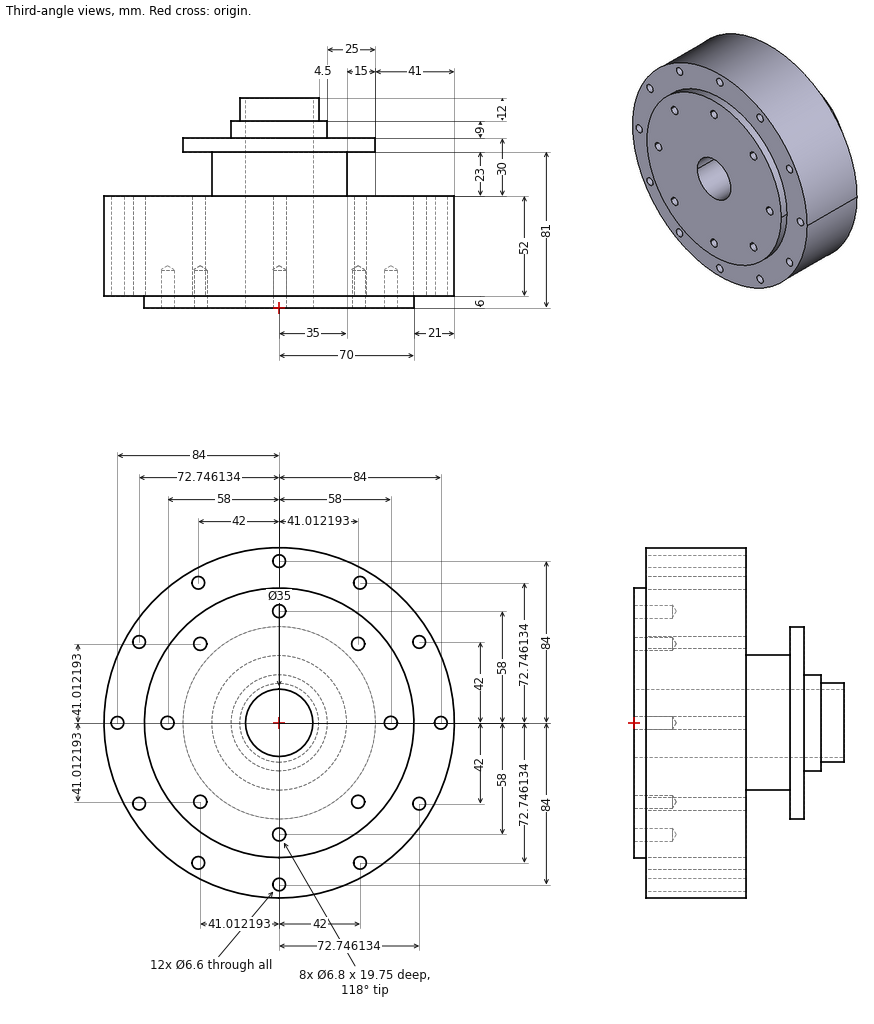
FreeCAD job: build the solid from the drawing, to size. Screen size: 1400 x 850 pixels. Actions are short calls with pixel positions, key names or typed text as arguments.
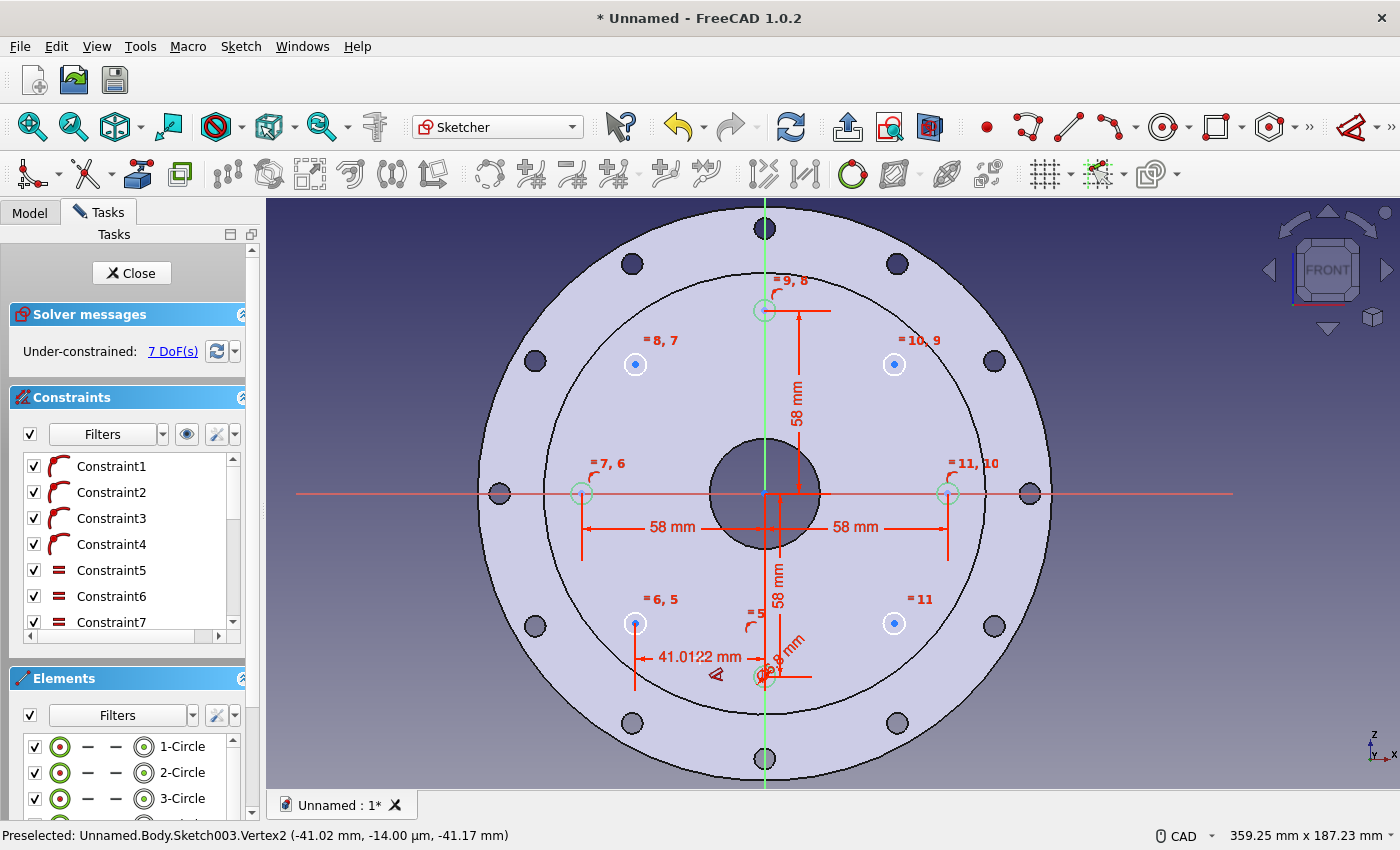
click(635, 624)
click(601, 559)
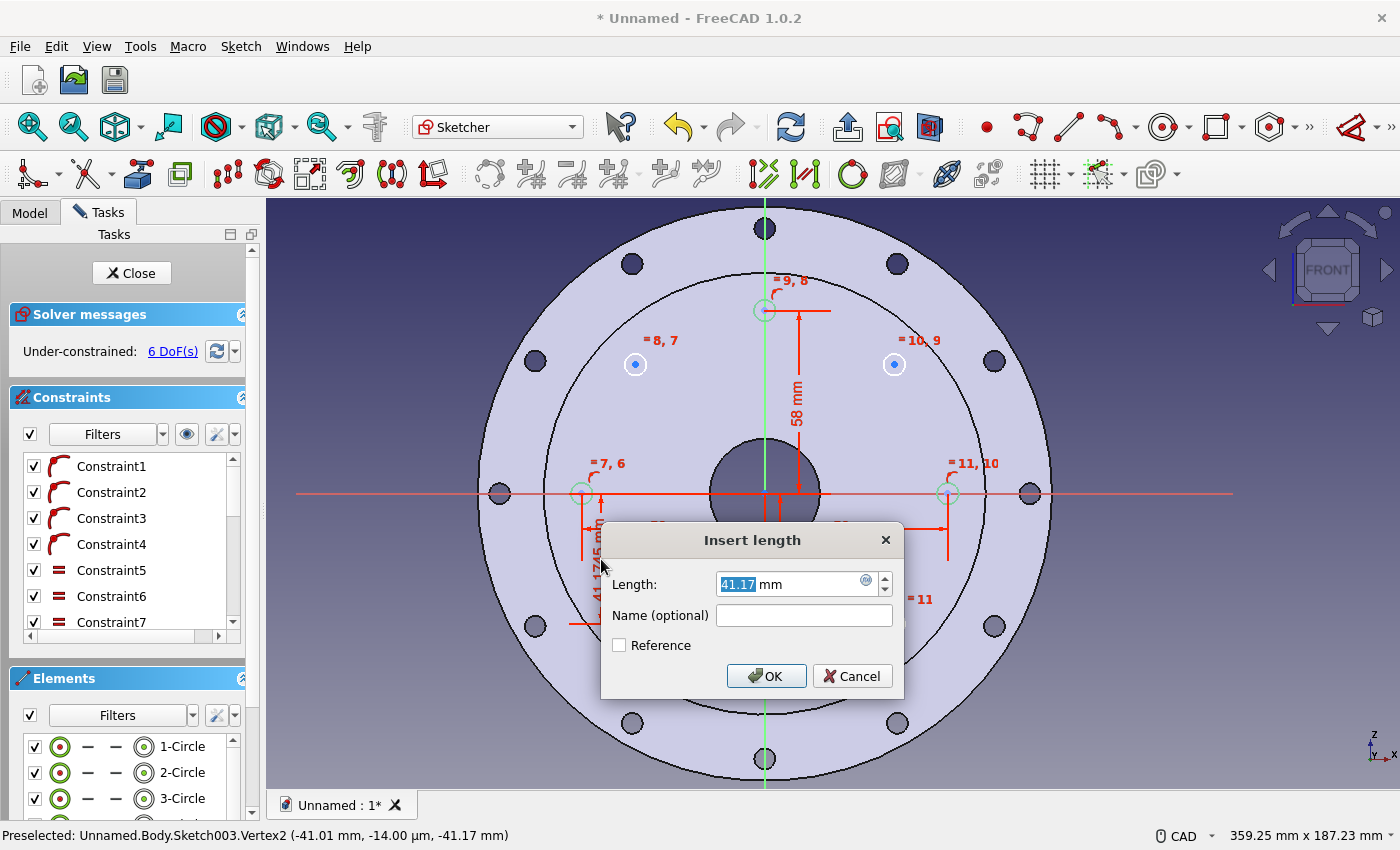
text(41.012193)
key(Return)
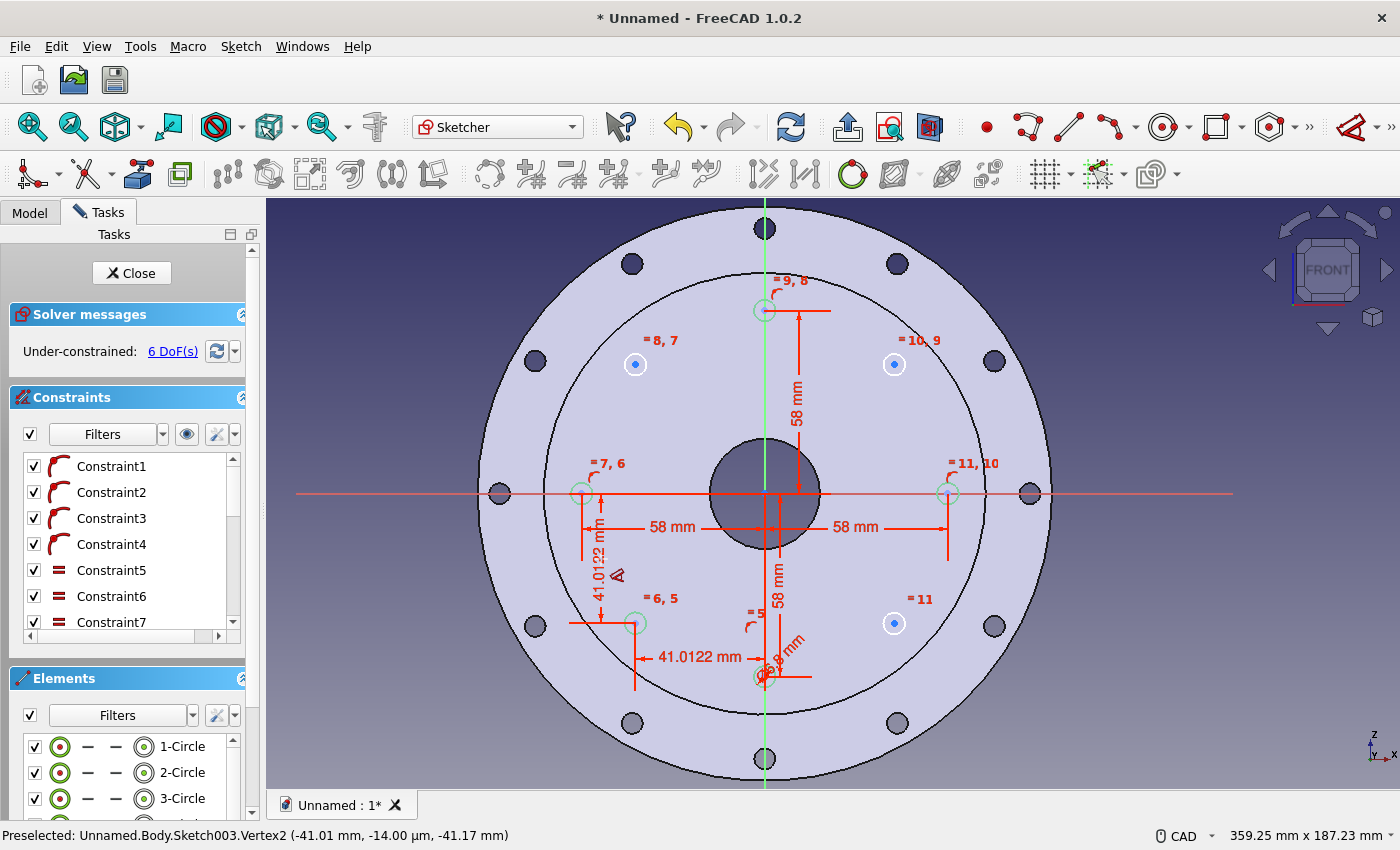
click(636, 365)
click(700, 331)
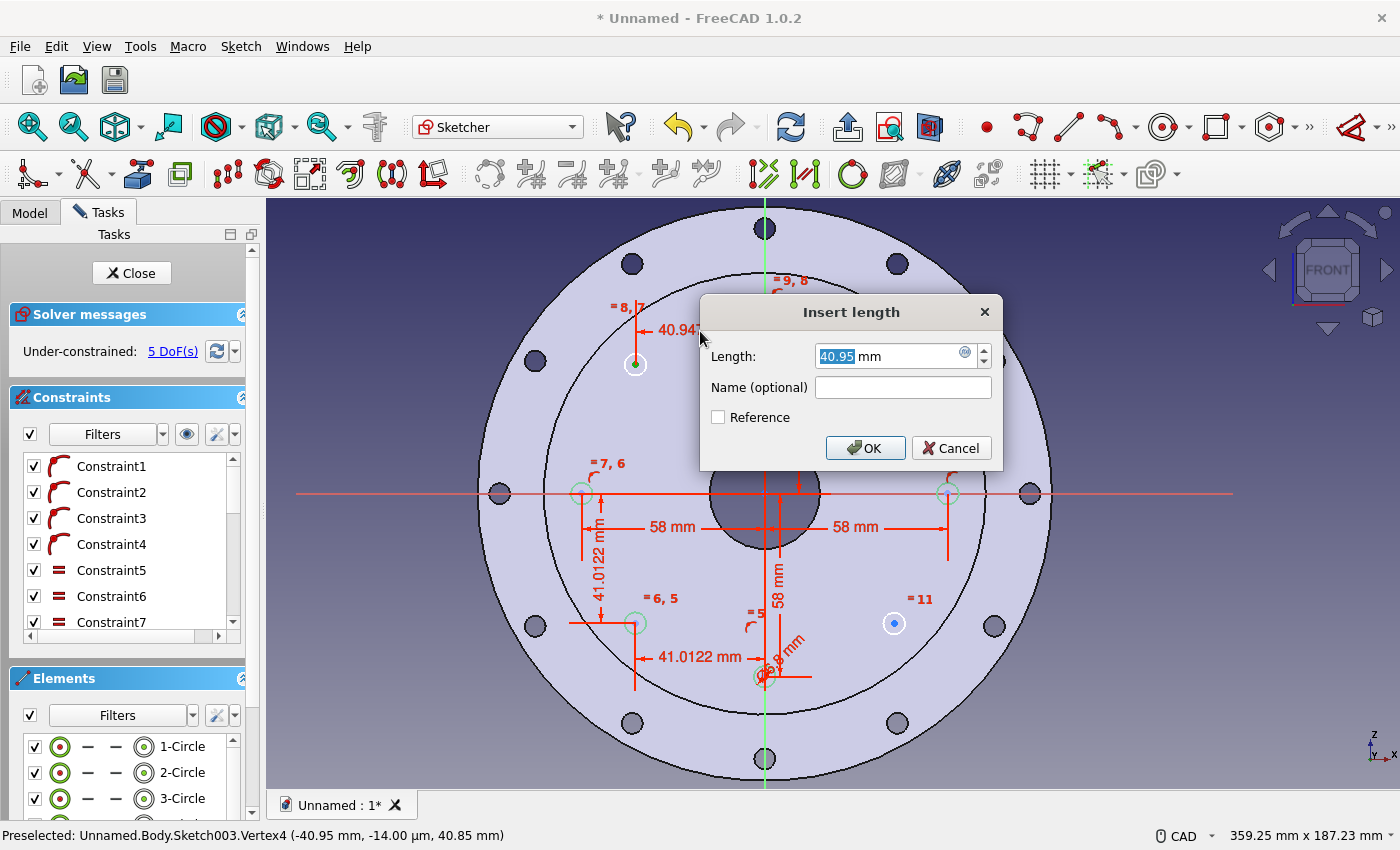
text(41.012193)
key(Return)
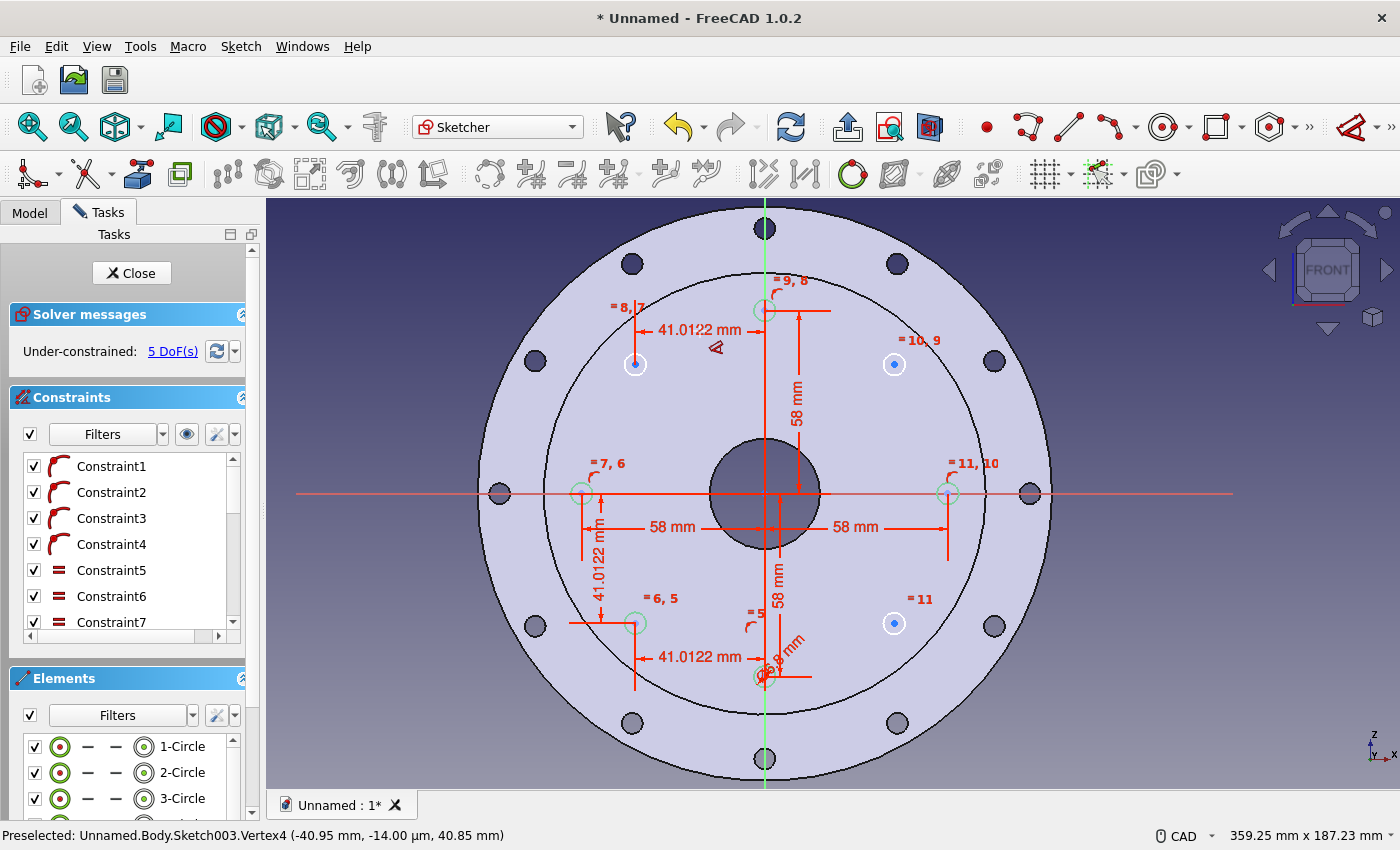
click(635, 365)
click(601, 429)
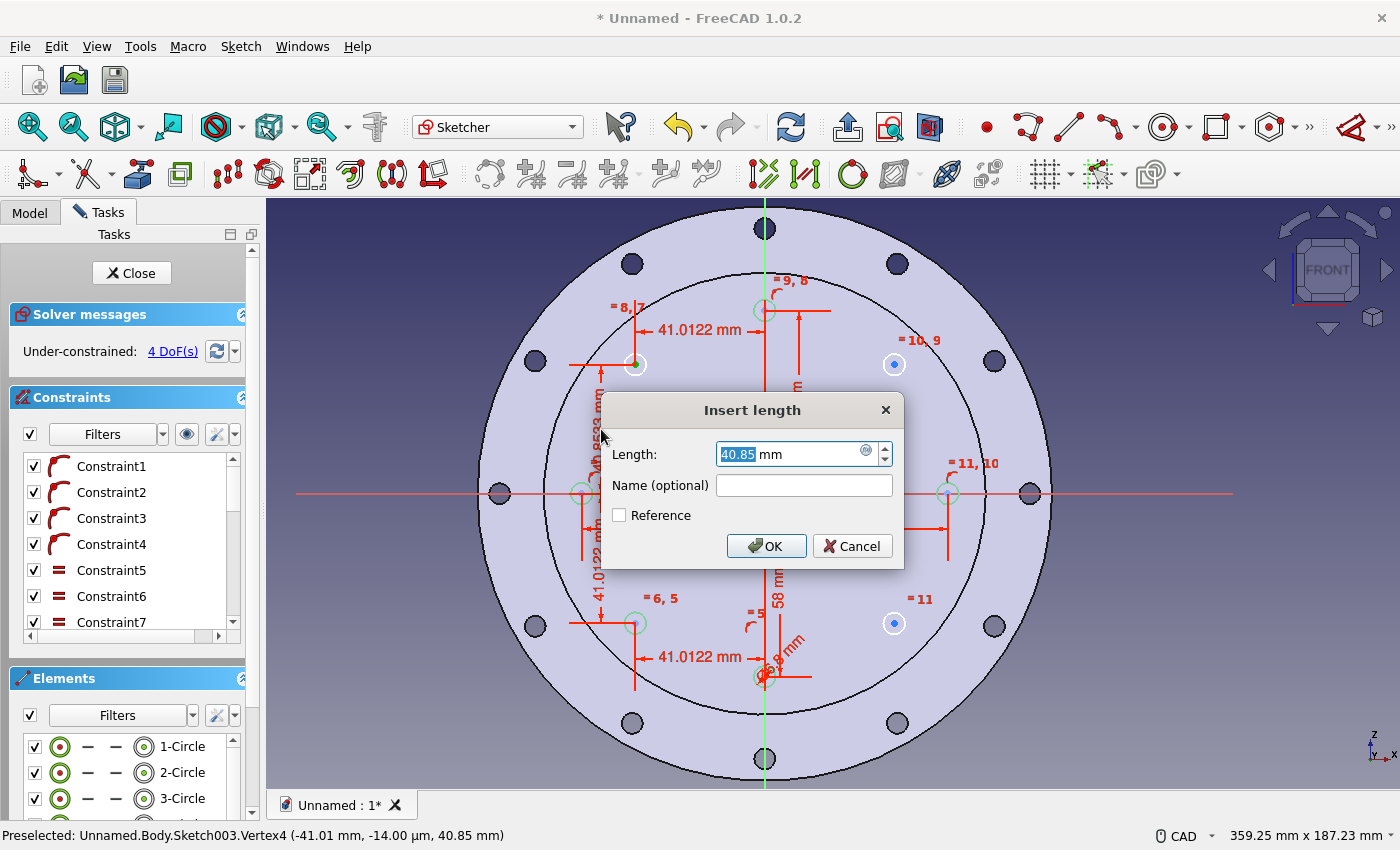
text(41.012193)
key(Return)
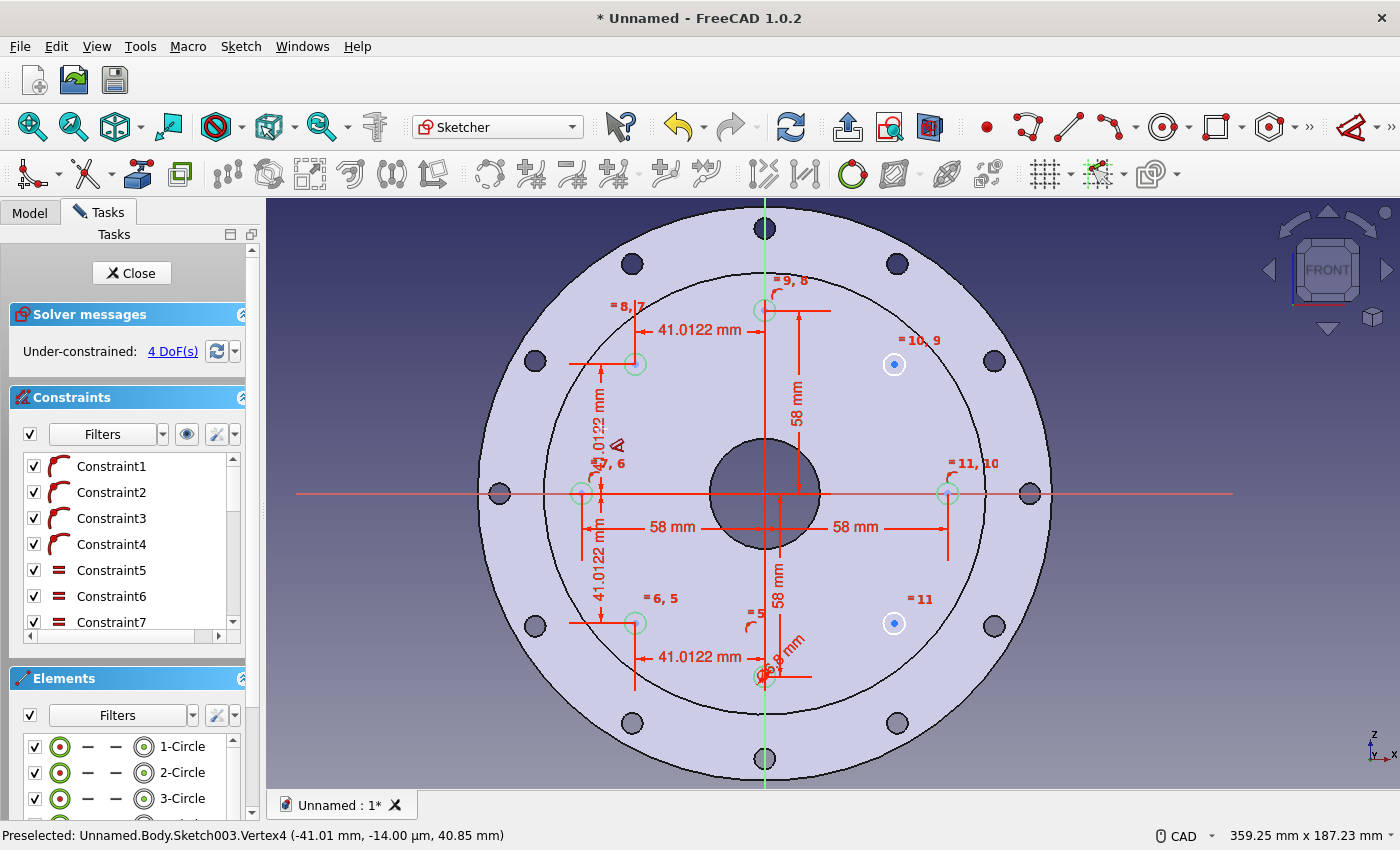
click(894, 365)
click(830, 331)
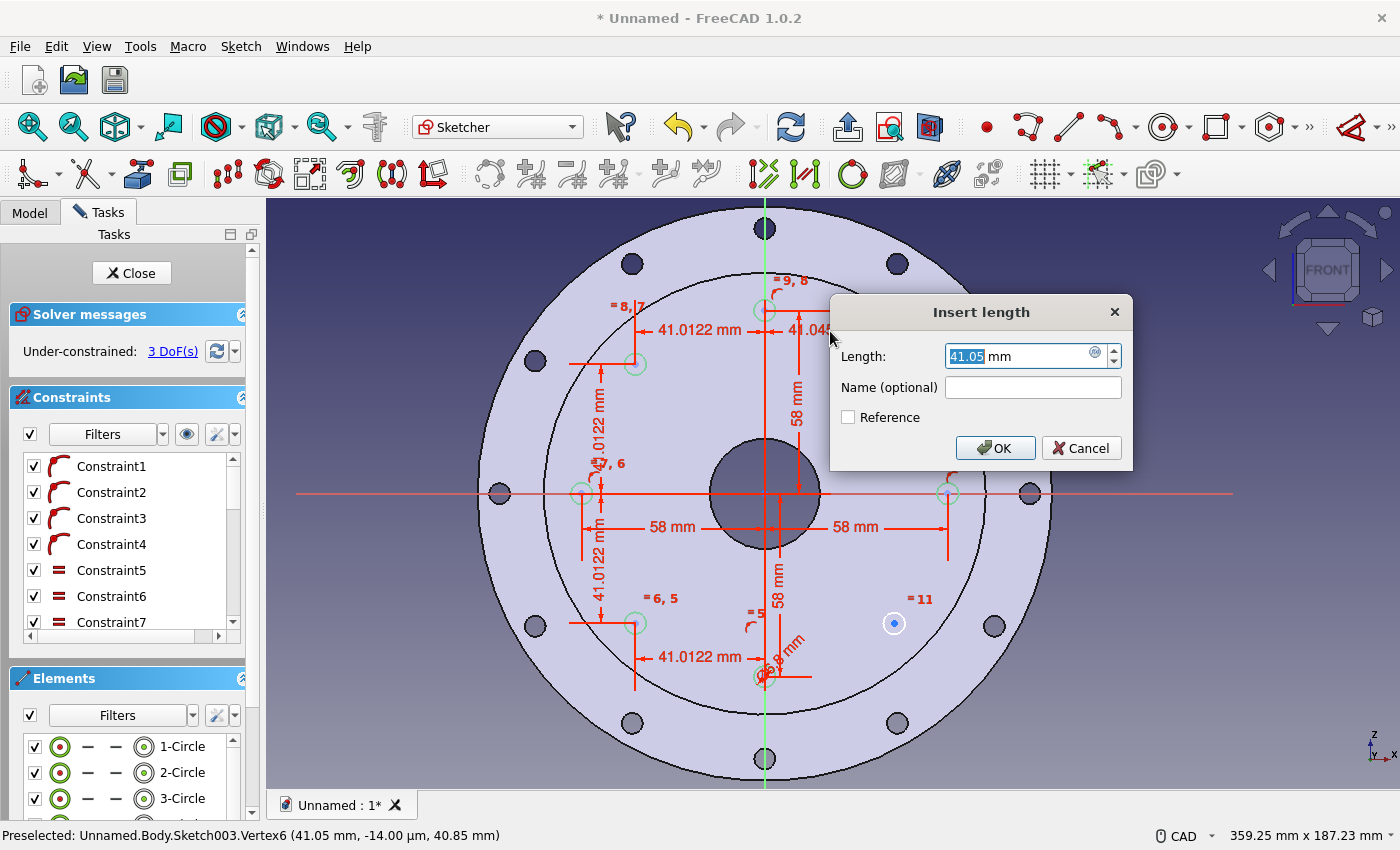
text(41.012193)
key(Return)